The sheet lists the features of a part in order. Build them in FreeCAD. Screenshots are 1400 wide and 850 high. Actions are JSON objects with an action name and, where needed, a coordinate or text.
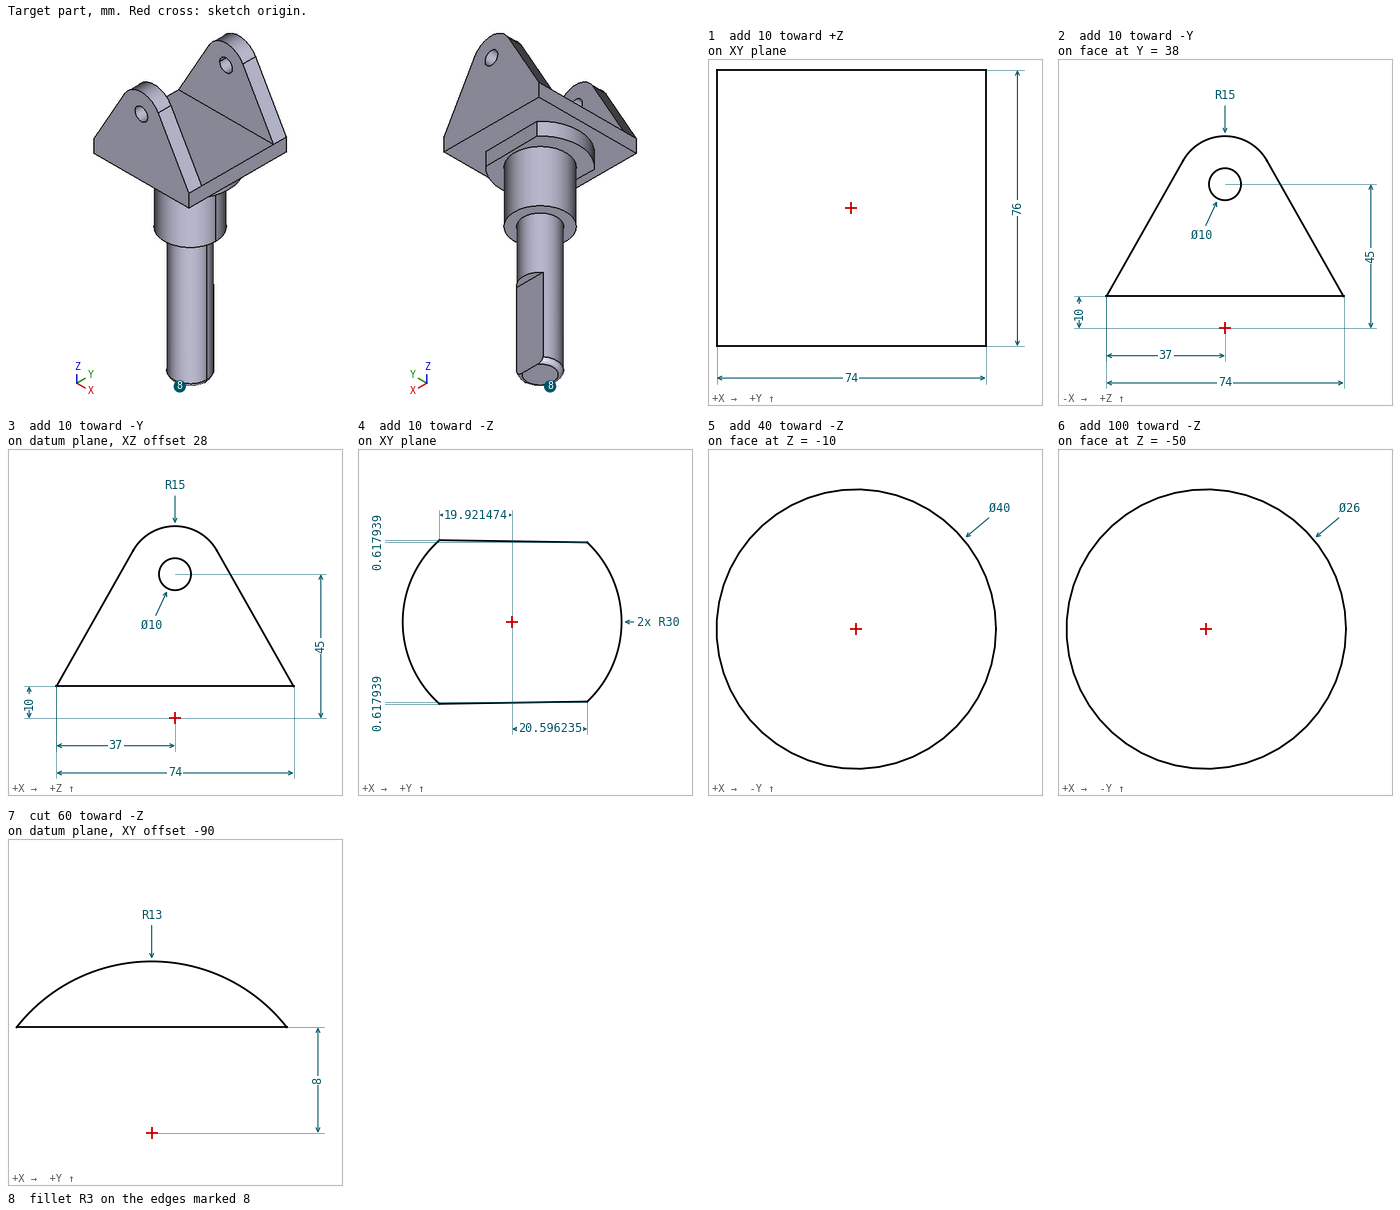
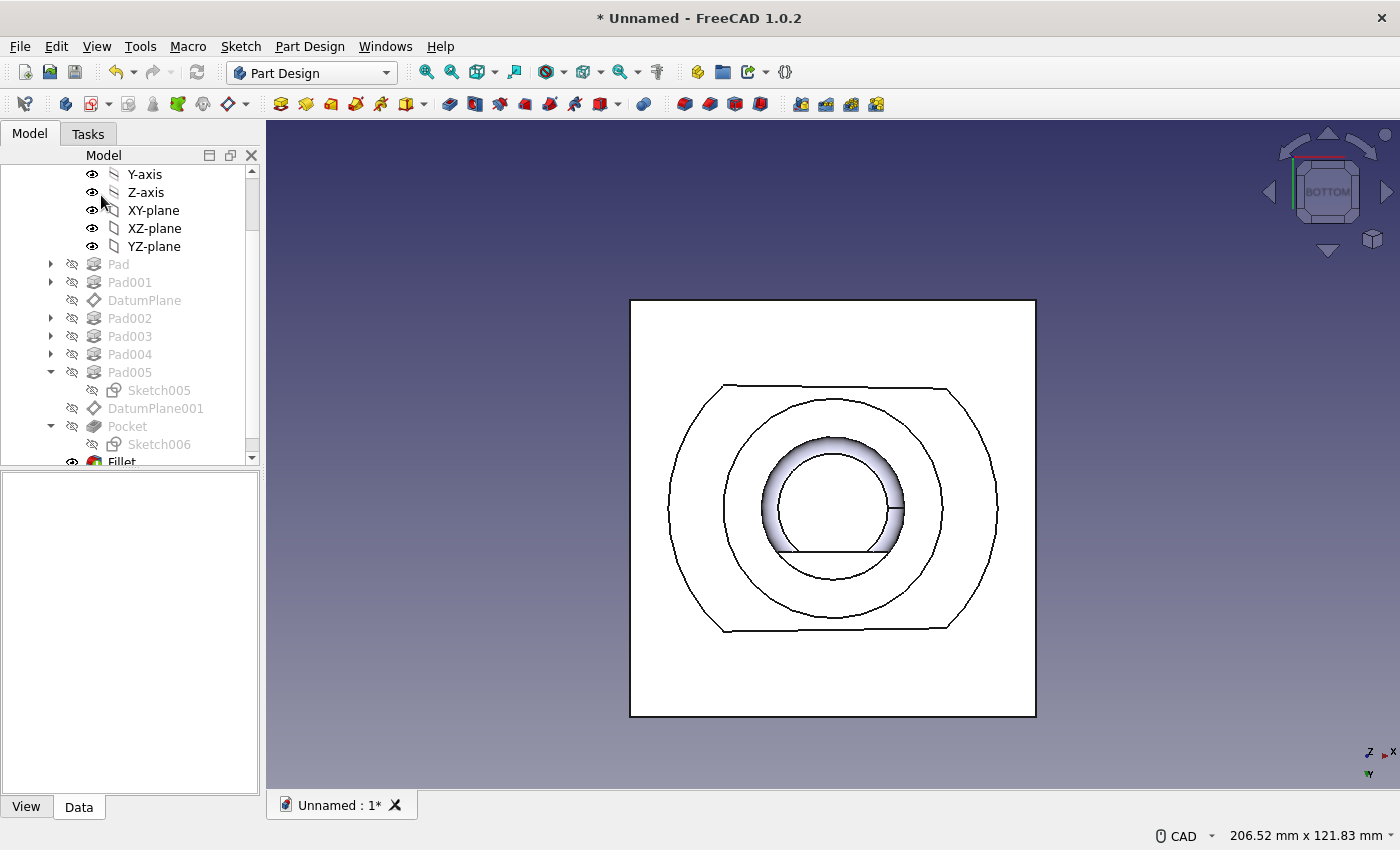
{"action": "key", "text": "0"}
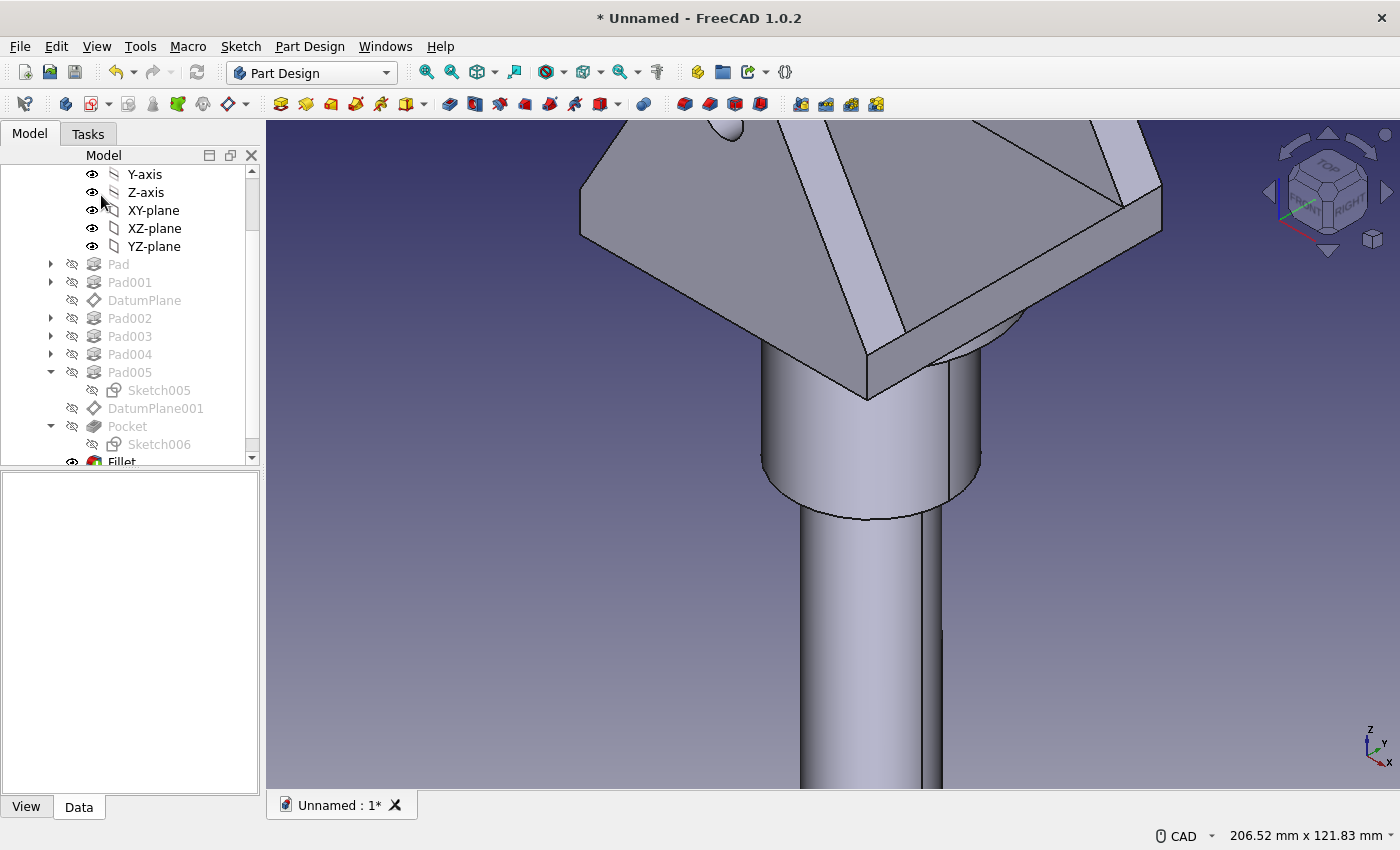
{"action": "left_click", "coordinate": [427, 72]}